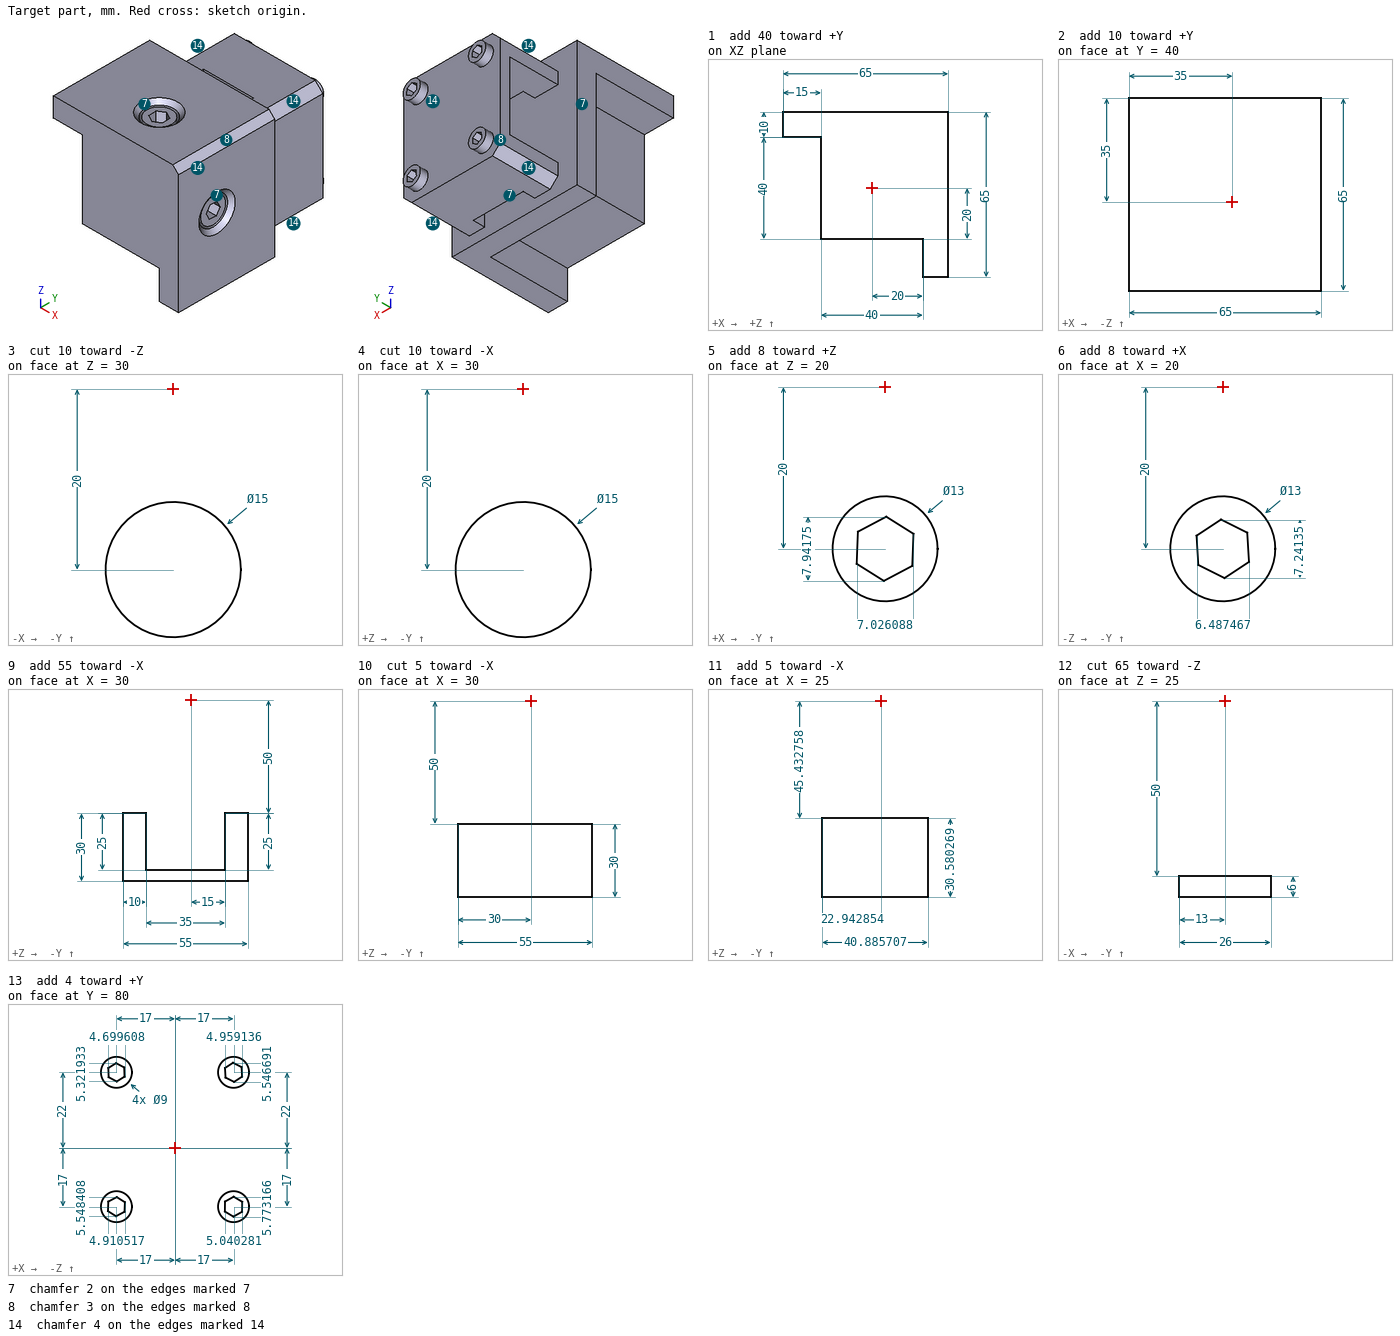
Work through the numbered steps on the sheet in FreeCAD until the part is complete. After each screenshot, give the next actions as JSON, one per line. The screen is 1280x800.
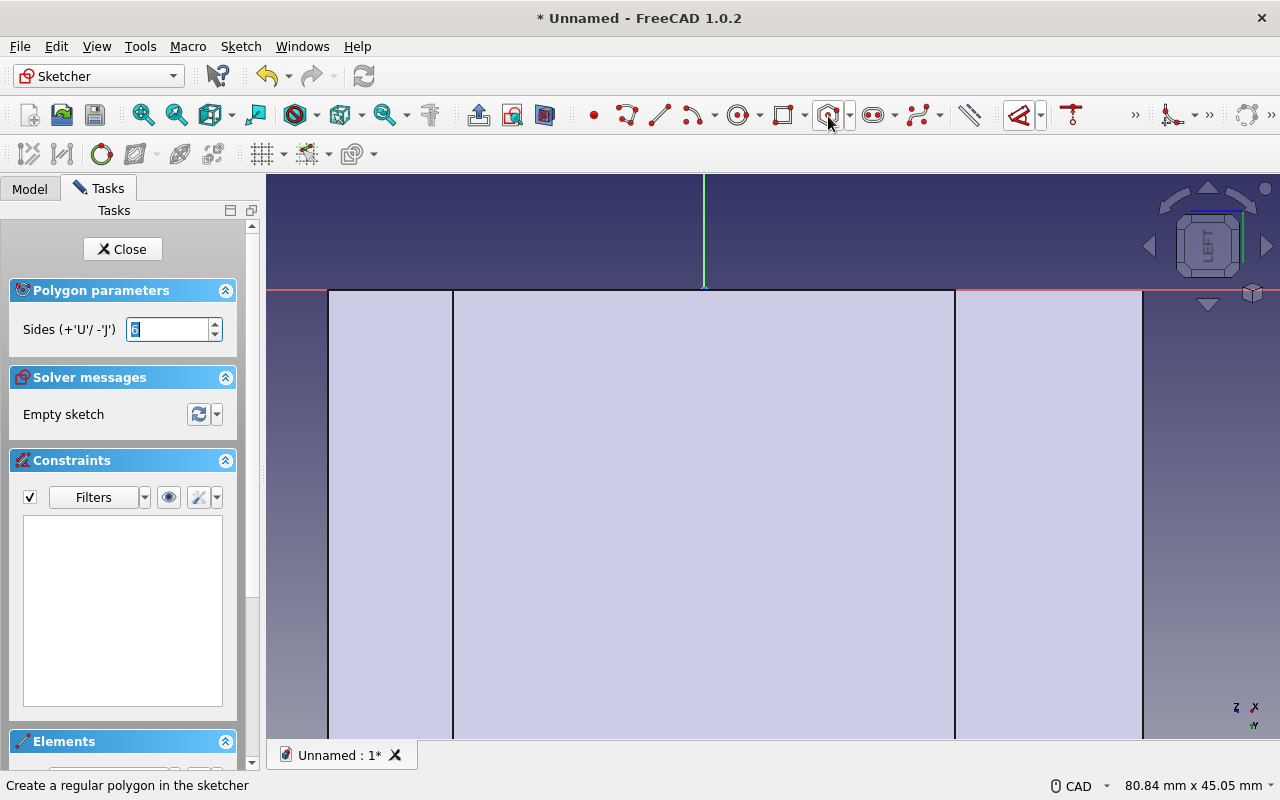
{"action": "left_click", "coordinate": [704, 541]}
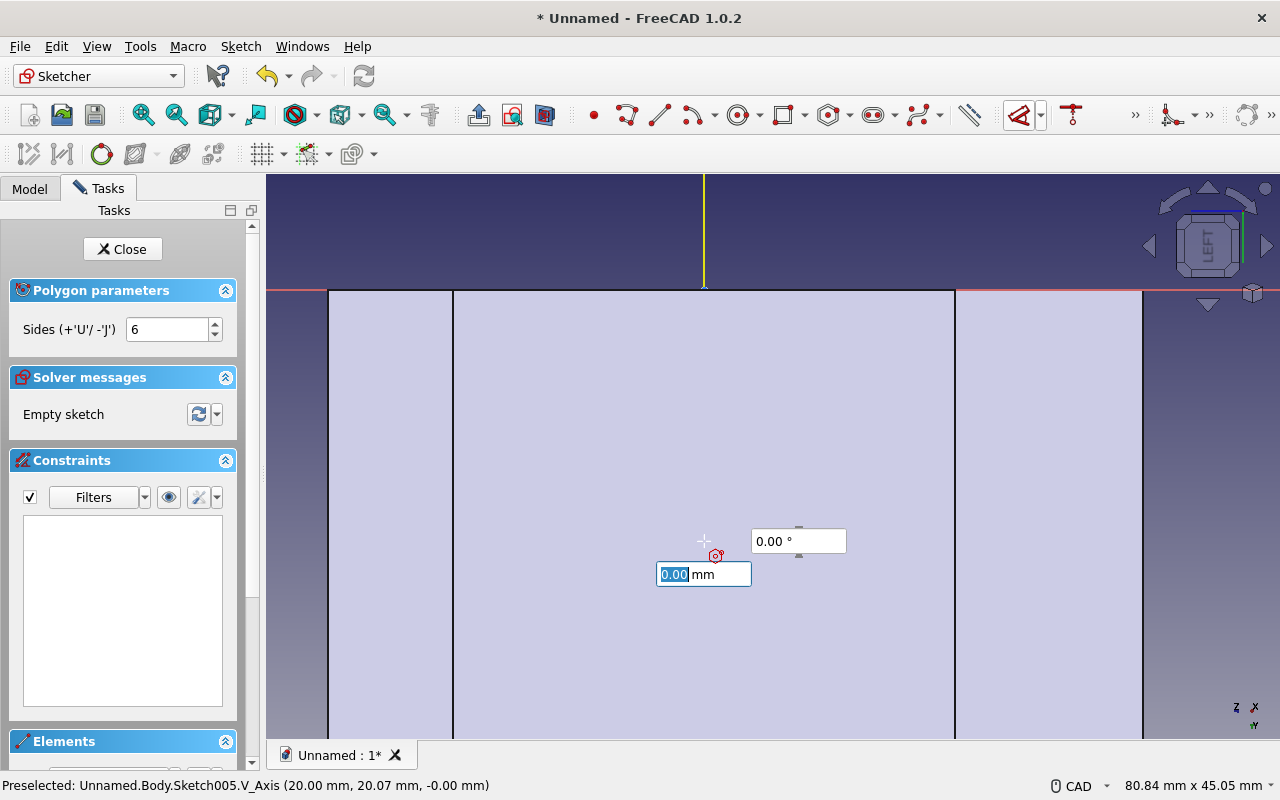
{"action": "left_click", "coordinate": [745, 561]}
{"action": "right_click", "coordinate": [745, 561]}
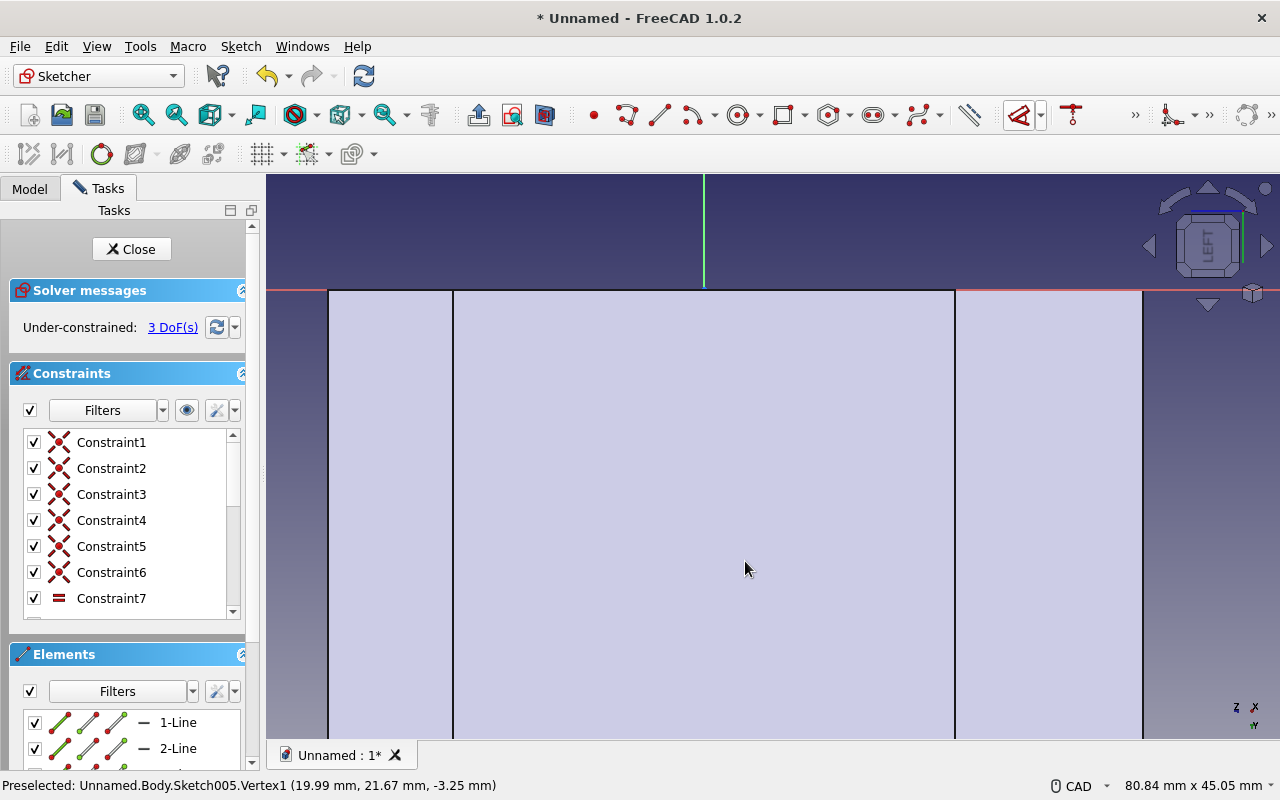
{"action": "left_click", "coordinate": [738, 116]}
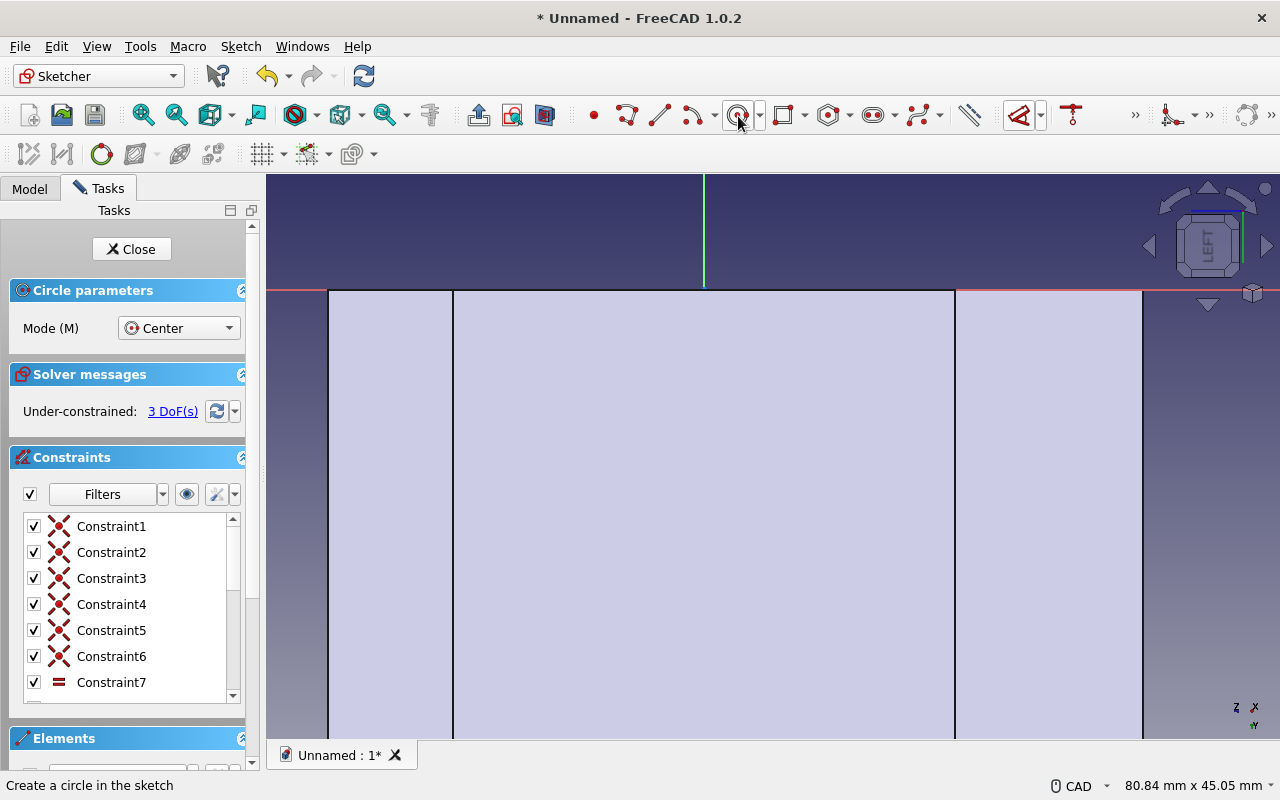
{"action": "left_click", "coordinate": [704, 542]}
{"action": "mouse_move", "coordinate": [762, 483]}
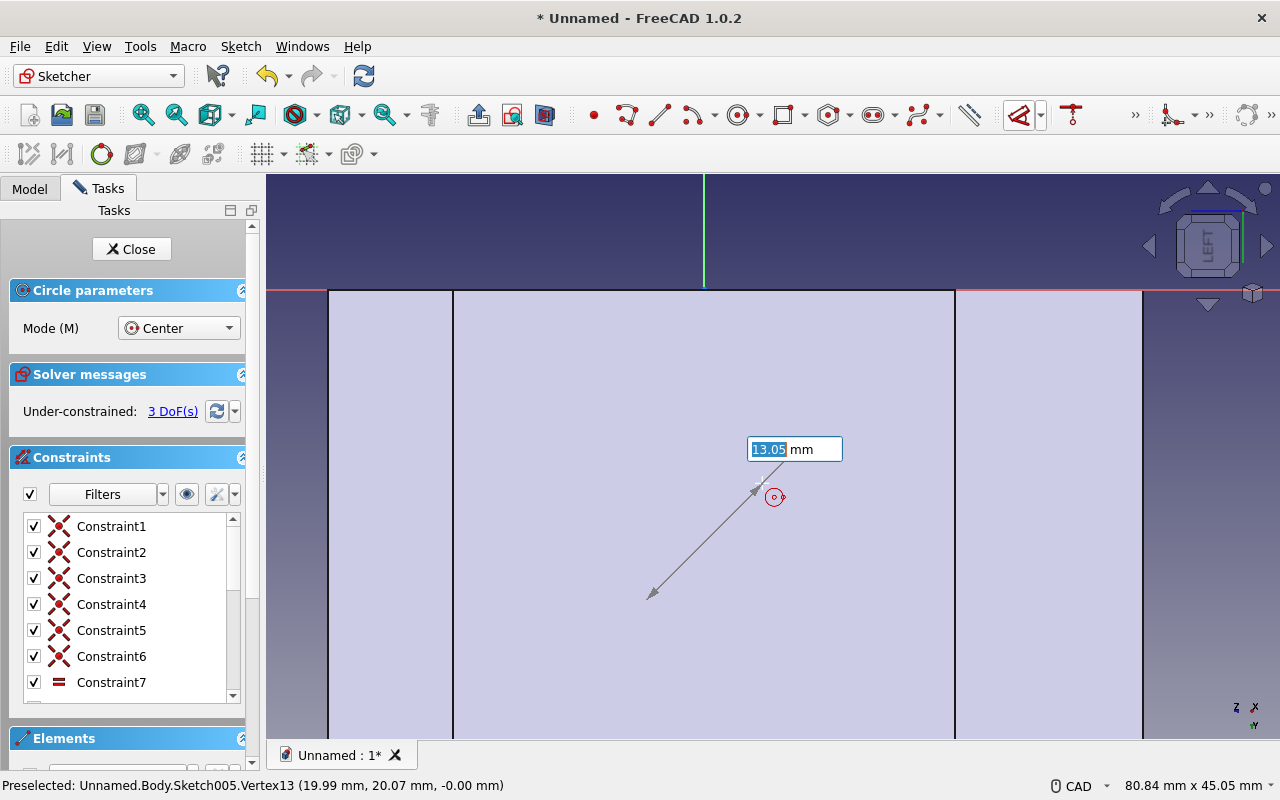
{"action": "type", "text": "13"}
{"action": "key", "text": "Return"}
{"action": "key", "text": "Escape"}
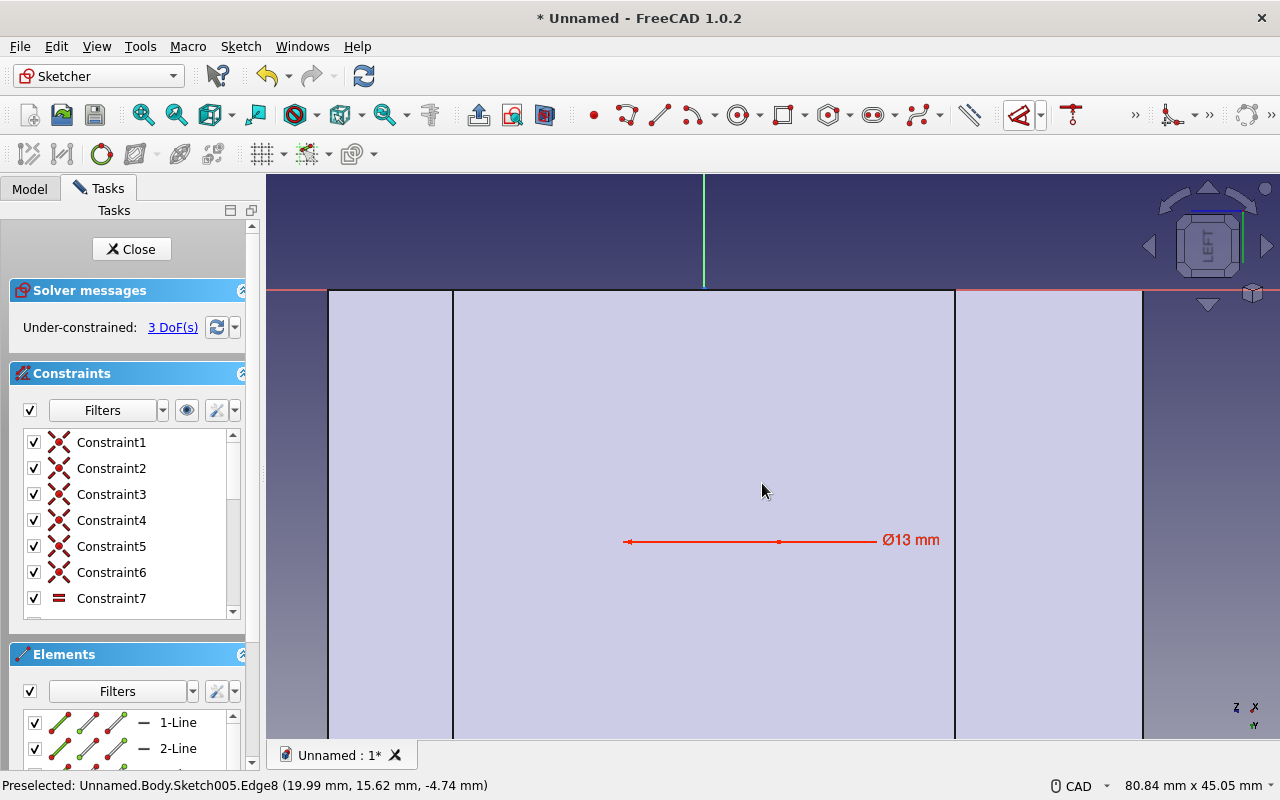
{"action": "left_click", "coordinate": [704, 542]}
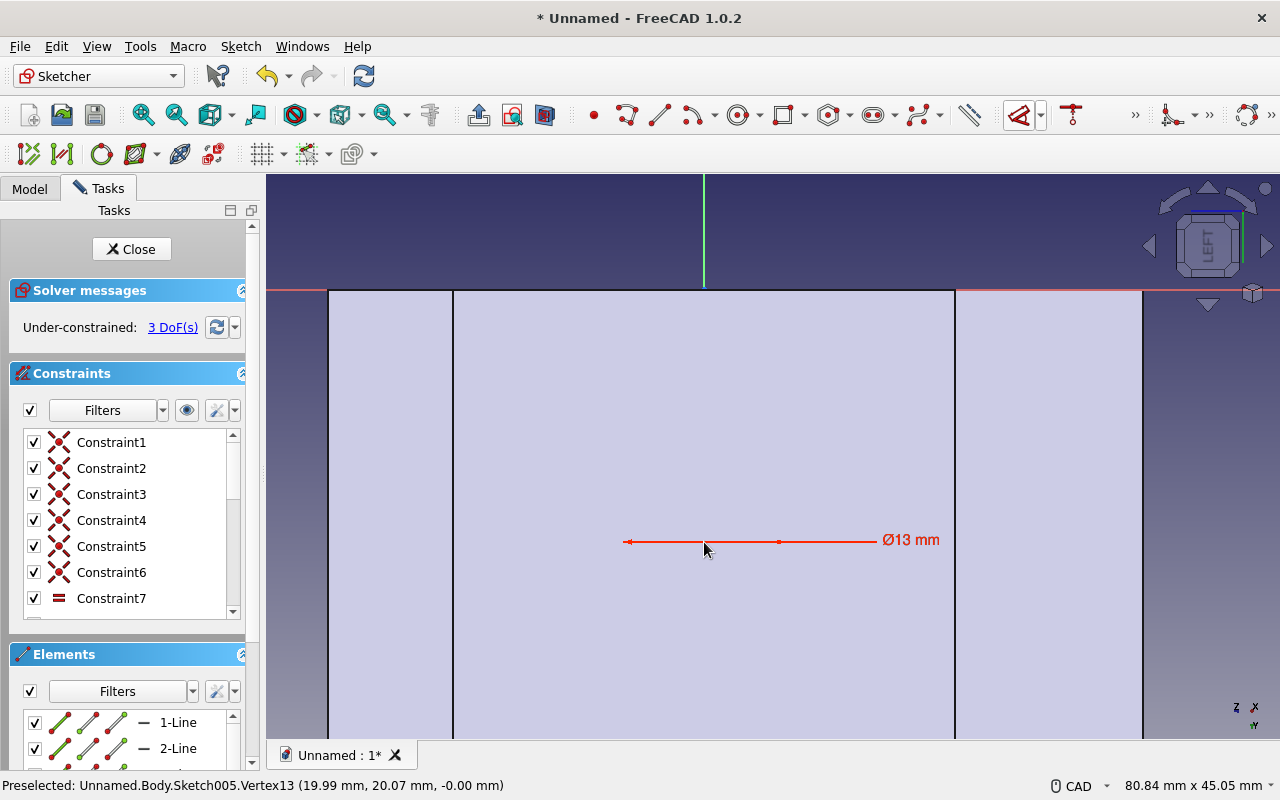
{"action": "left_click", "coordinate": [1040, 116]}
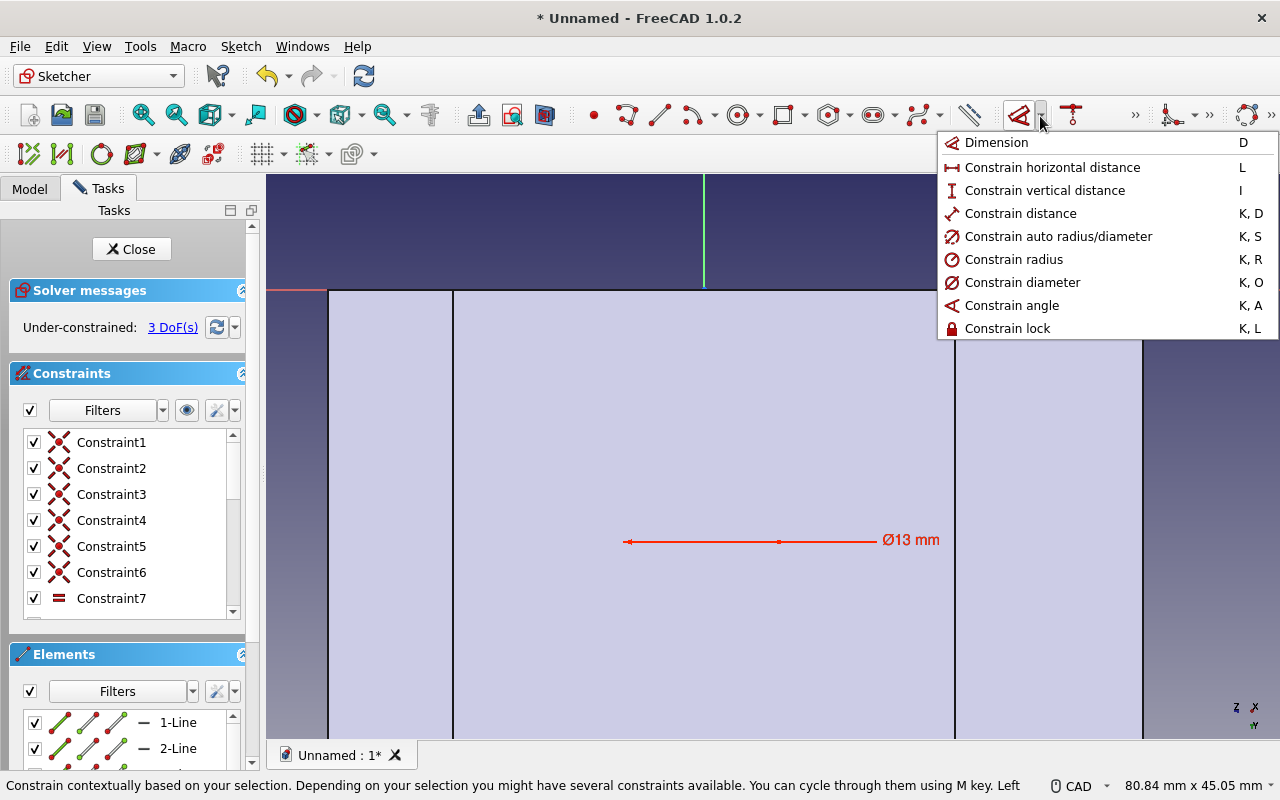
{"action": "left_click", "coordinate": [1108, 190]}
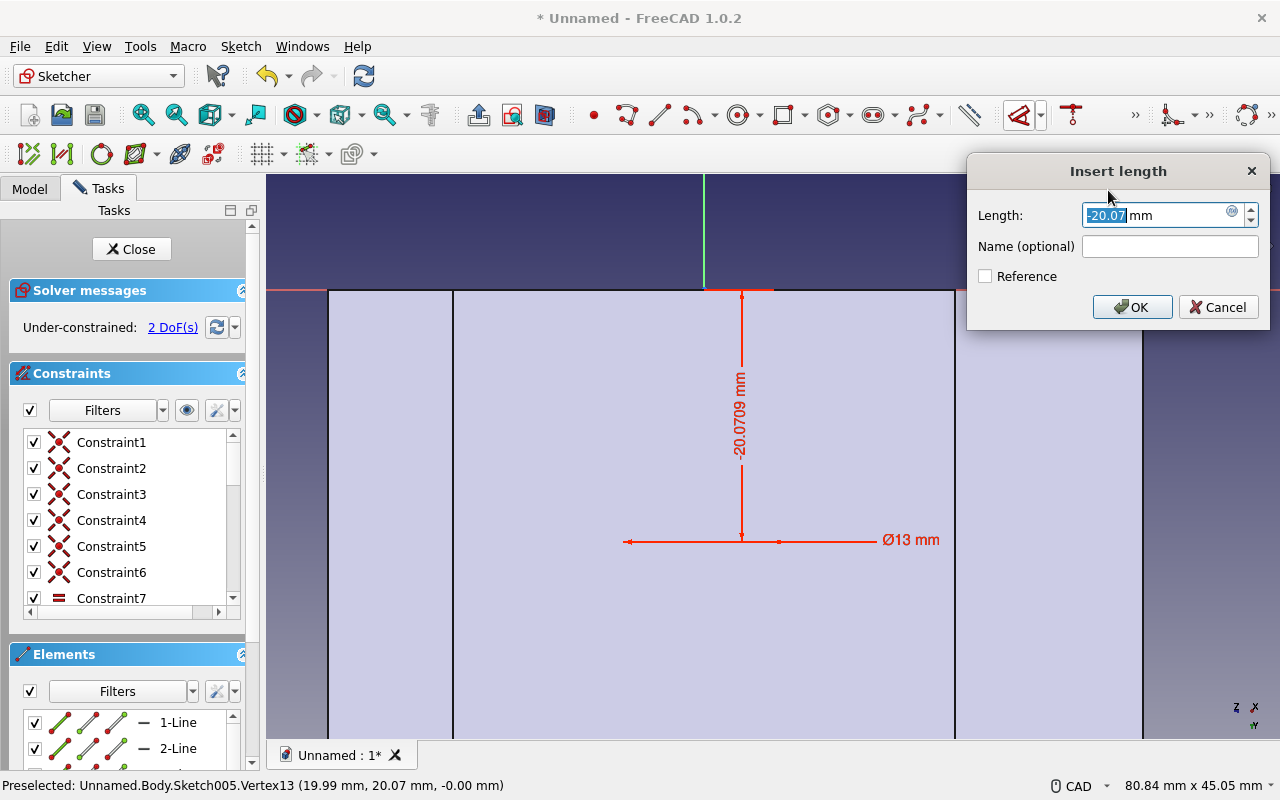
{"action": "type", "text": "-20"}
{"action": "key", "text": "Return"}